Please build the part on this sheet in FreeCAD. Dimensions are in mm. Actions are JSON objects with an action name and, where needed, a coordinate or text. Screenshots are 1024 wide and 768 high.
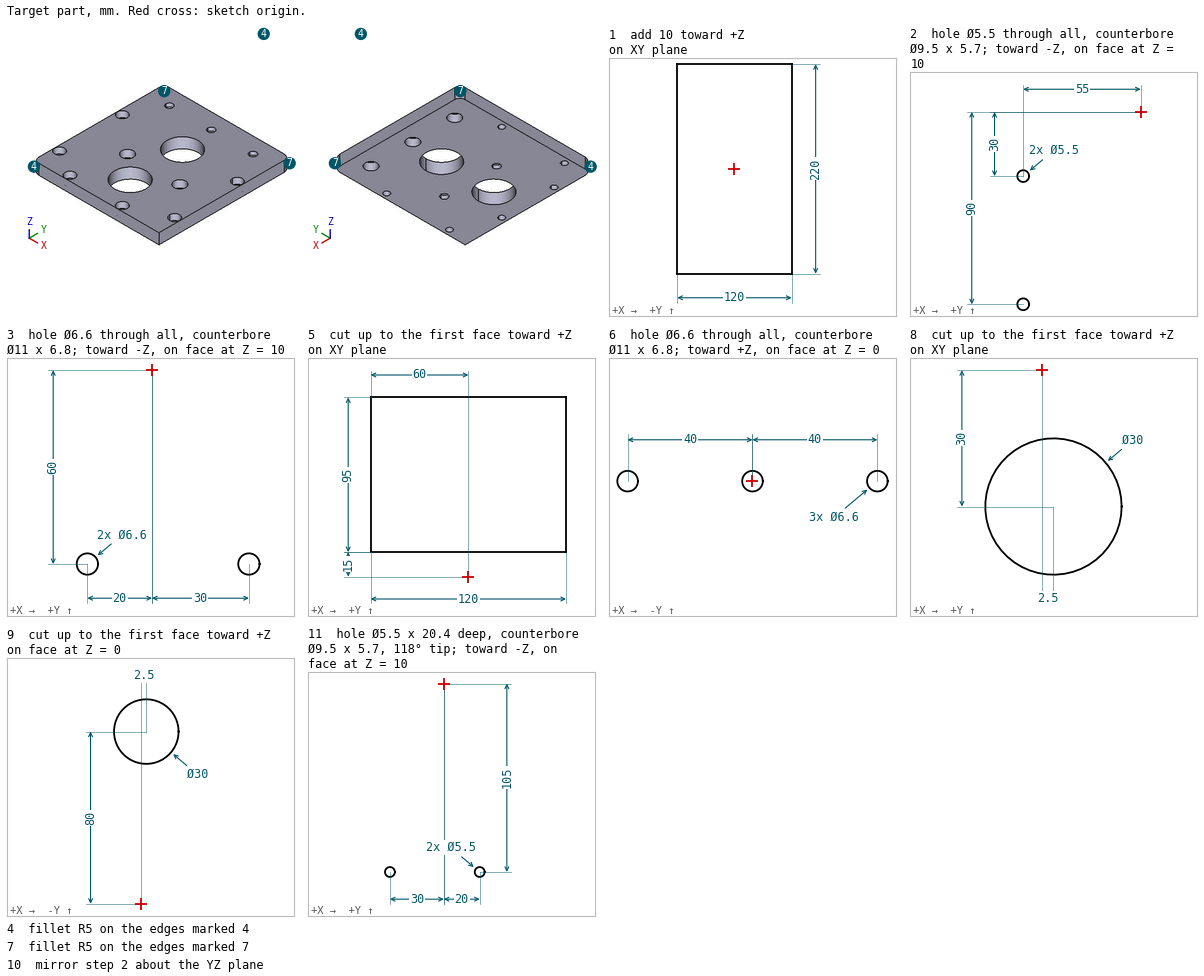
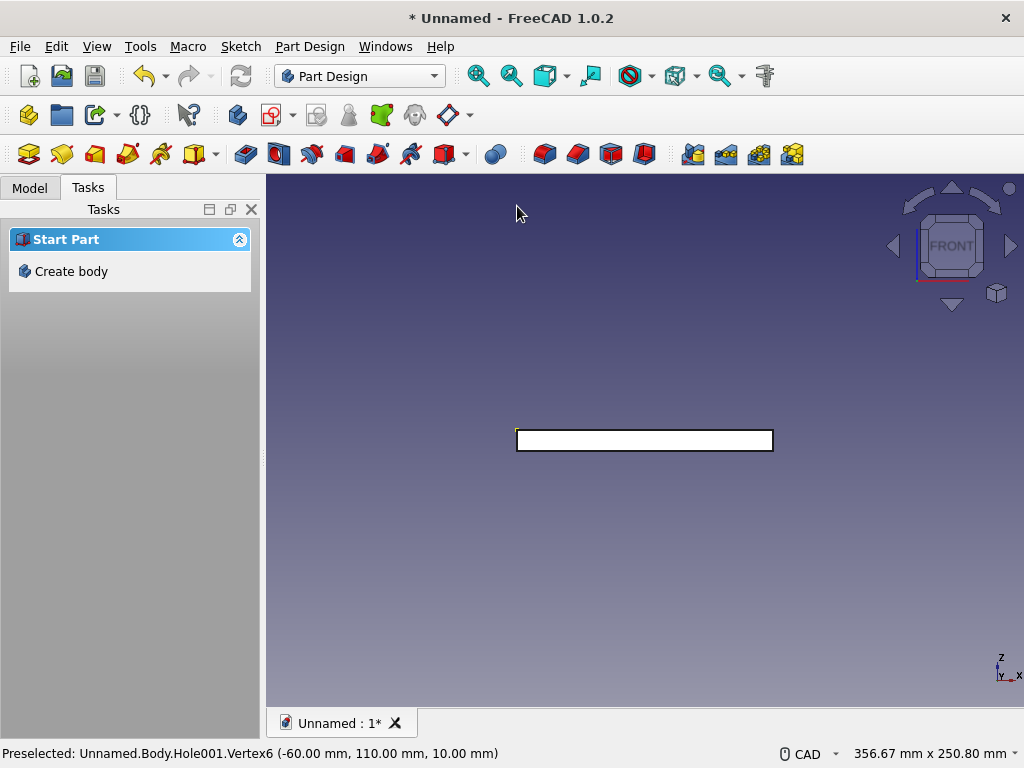
{"action": "left_click", "coordinate": [479, 76]}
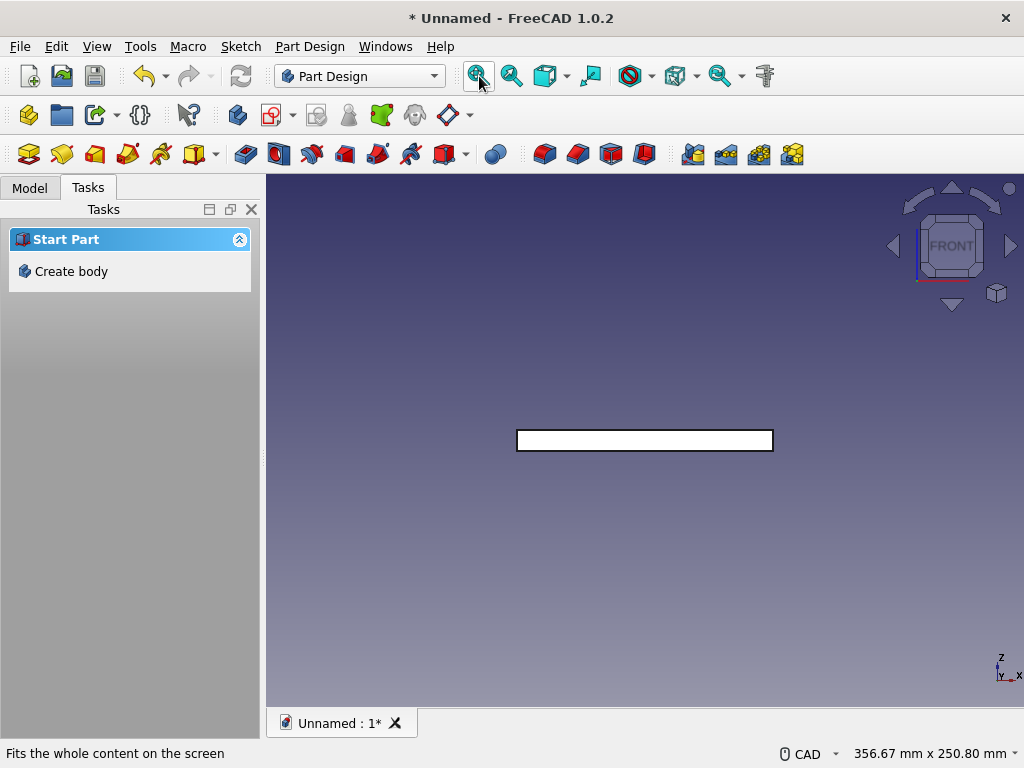
{"action": "left_click", "coordinate": [517, 440]}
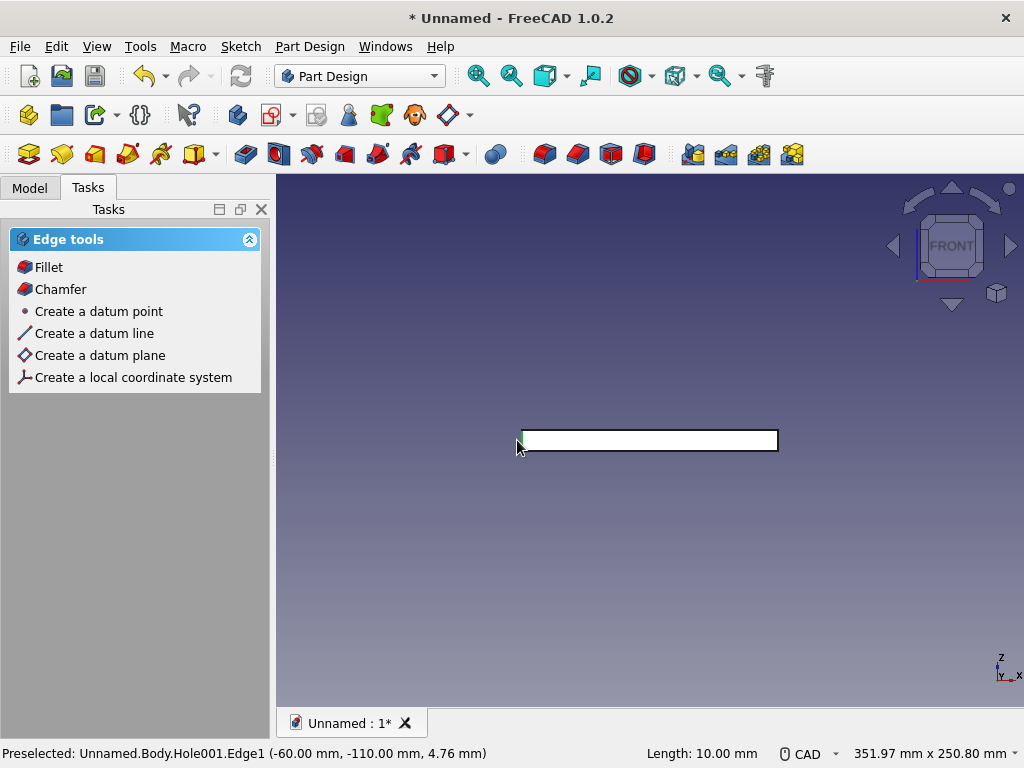
{"action": "scroll", "coordinate": [522, 440], "scroll_direction": "up", "scroll_amount": 4}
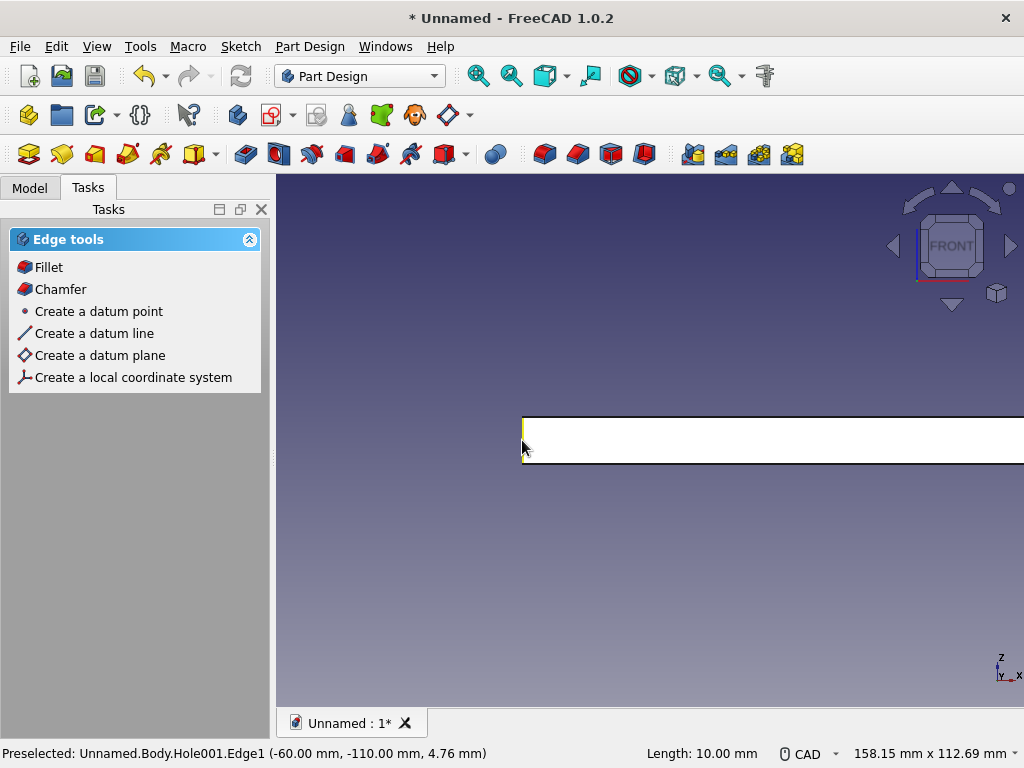
{"action": "left_click", "coordinate": [479, 76]}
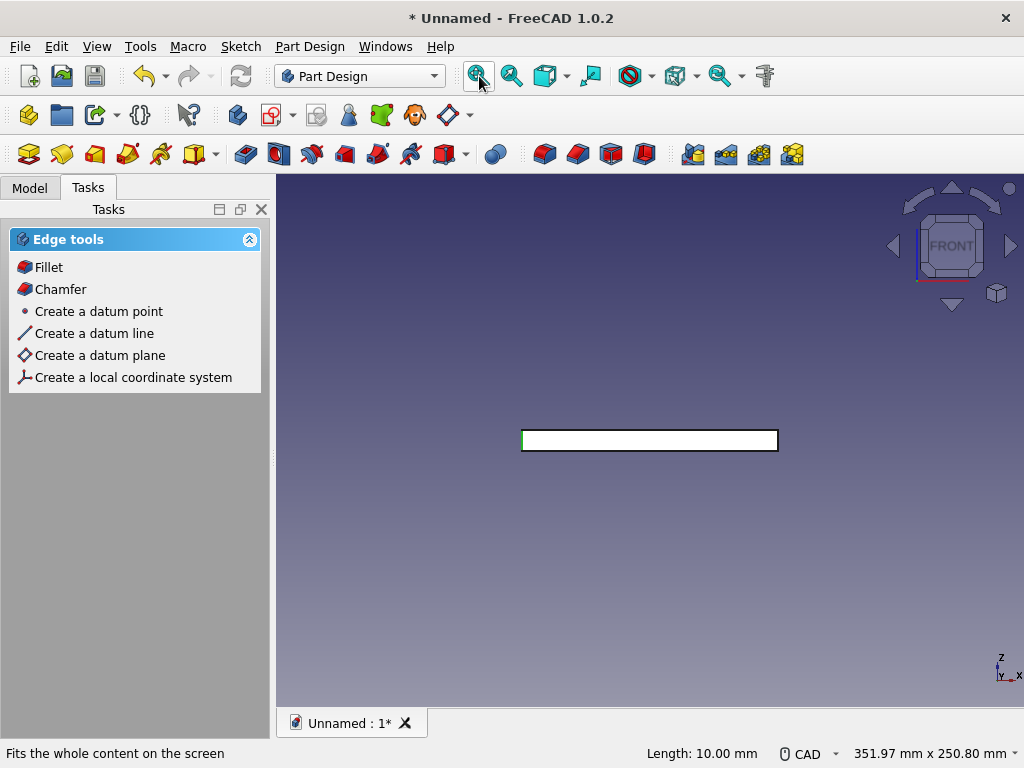
{"action": "key", "text": "3"}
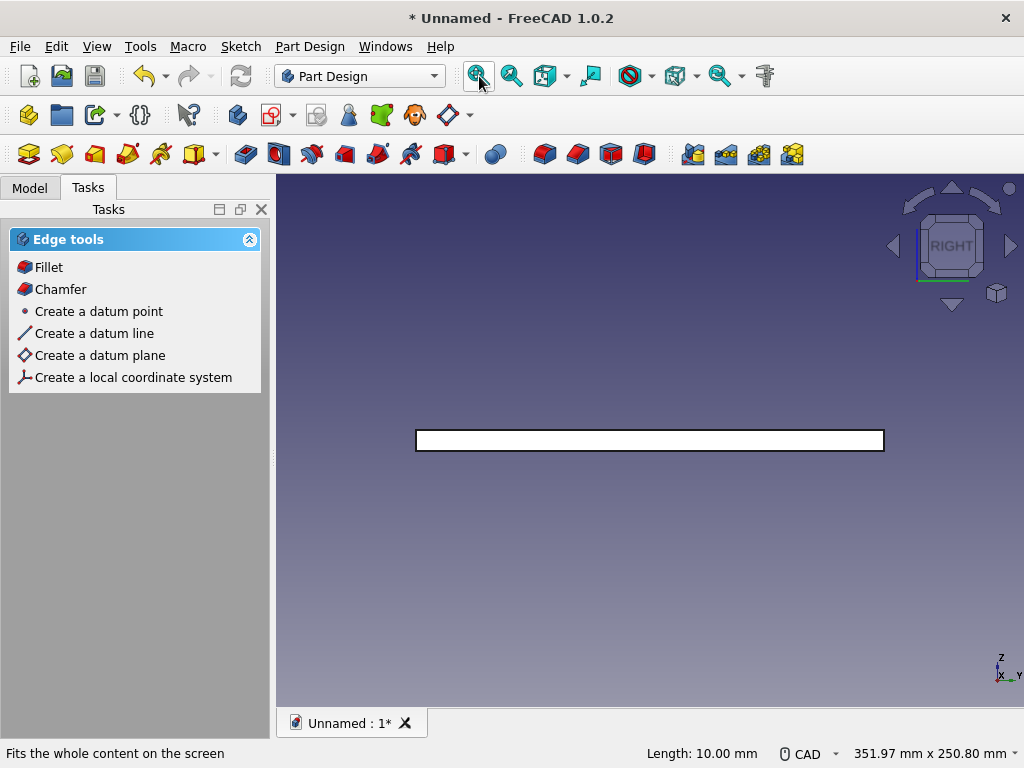
{"action": "key", "text": "5"}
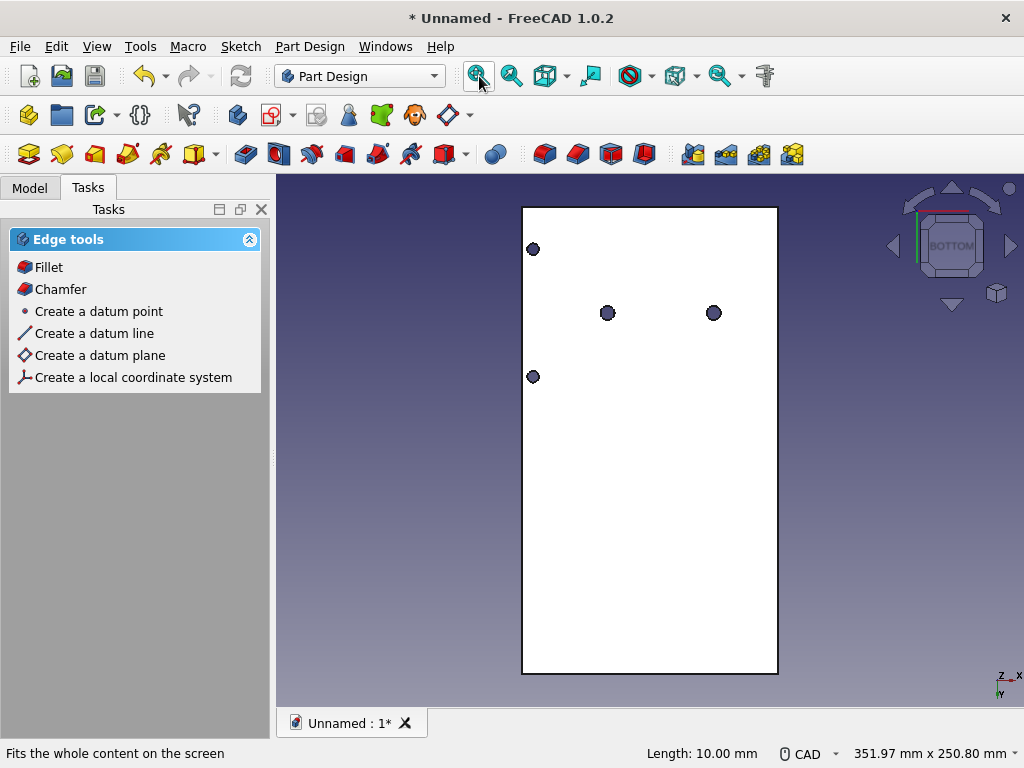
{"action": "scroll", "coordinate": [522, 673], "scroll_direction": "up", "scroll_amount": 4}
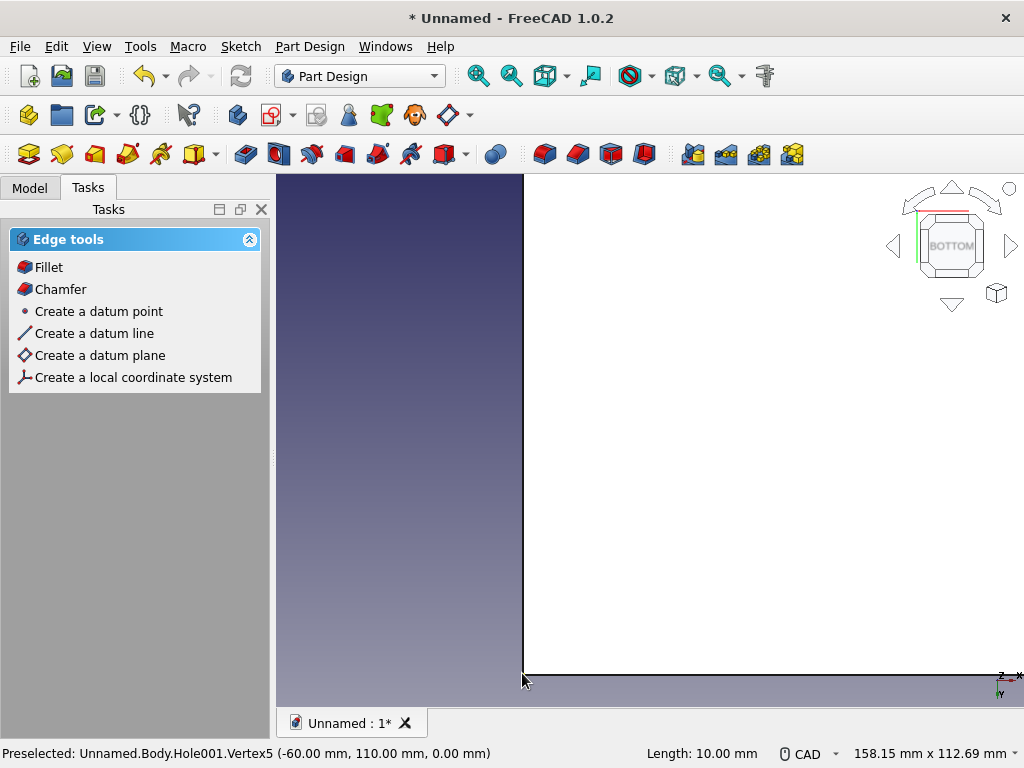
{"action": "left_click", "coordinate": [479, 76]}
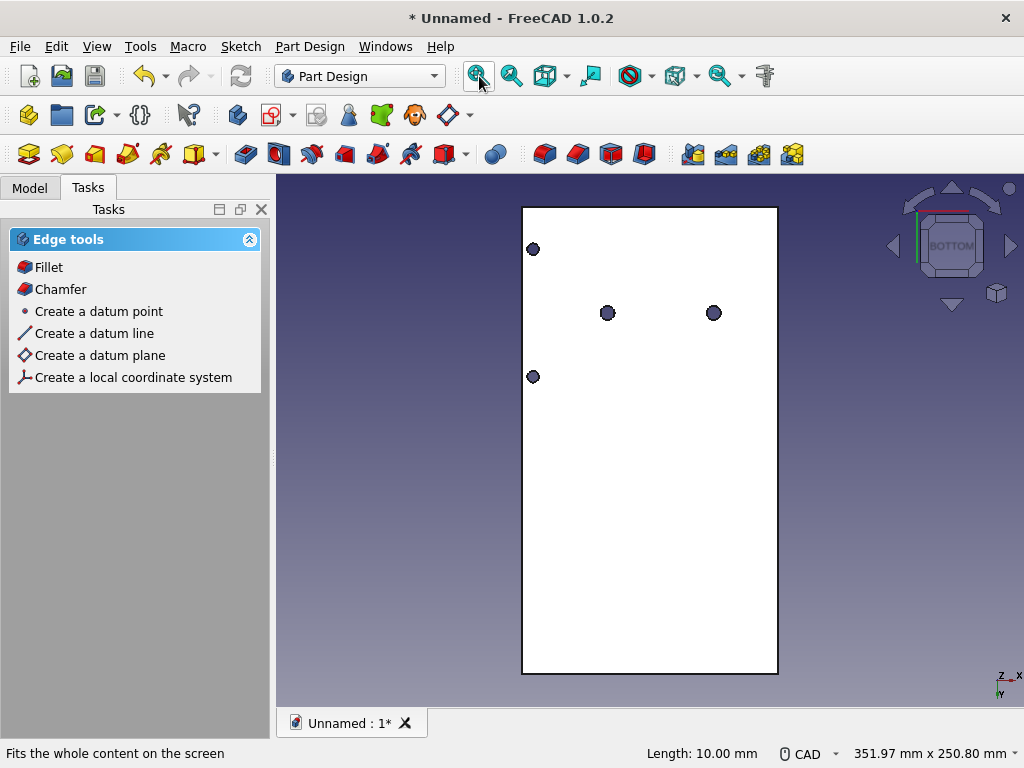
{"action": "key", "text": "4"}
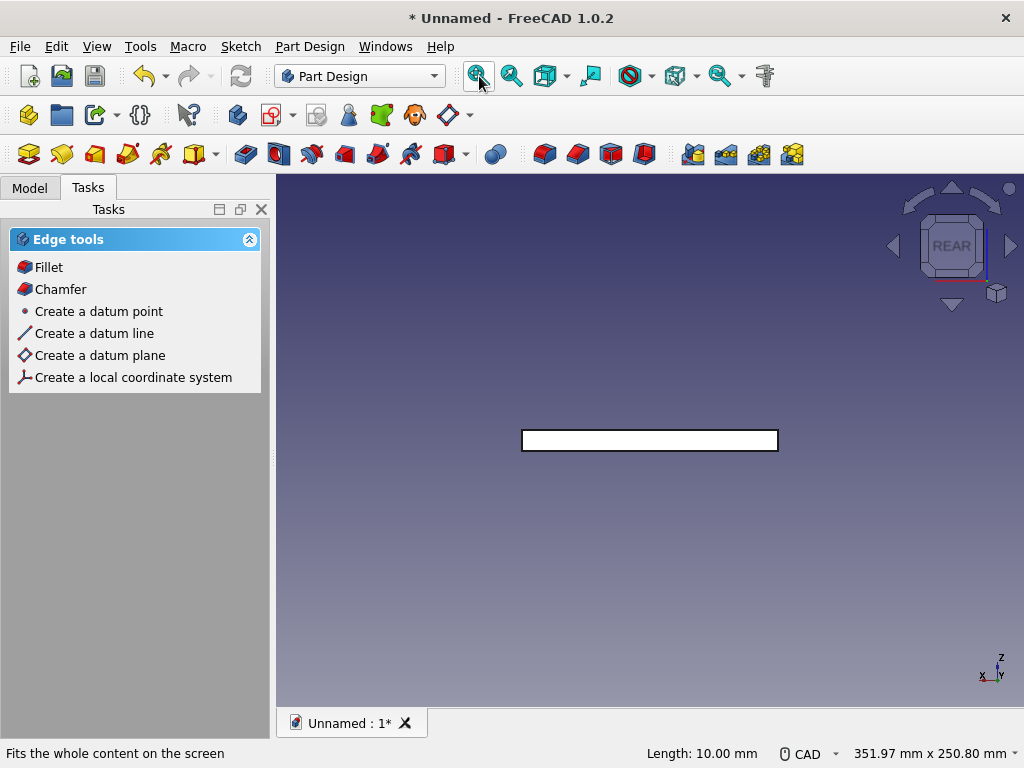
{"action": "left_click", "coordinate": [479, 76]}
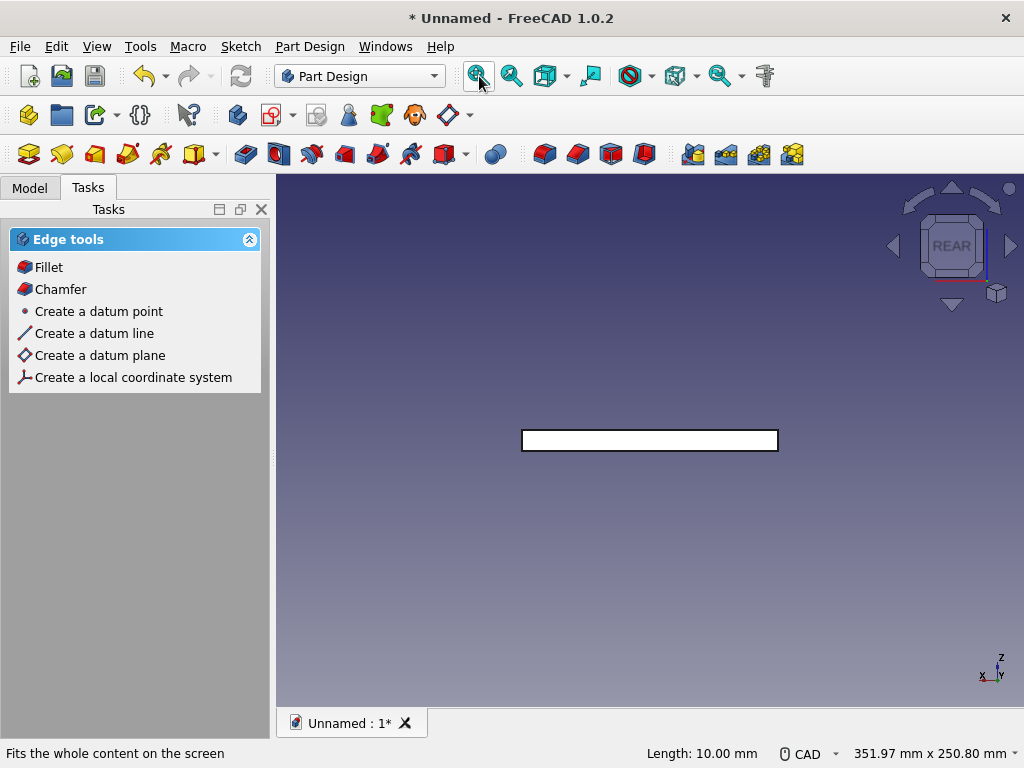
{"action": "left_click", "coordinate": [778, 440], "text": "ctrl"}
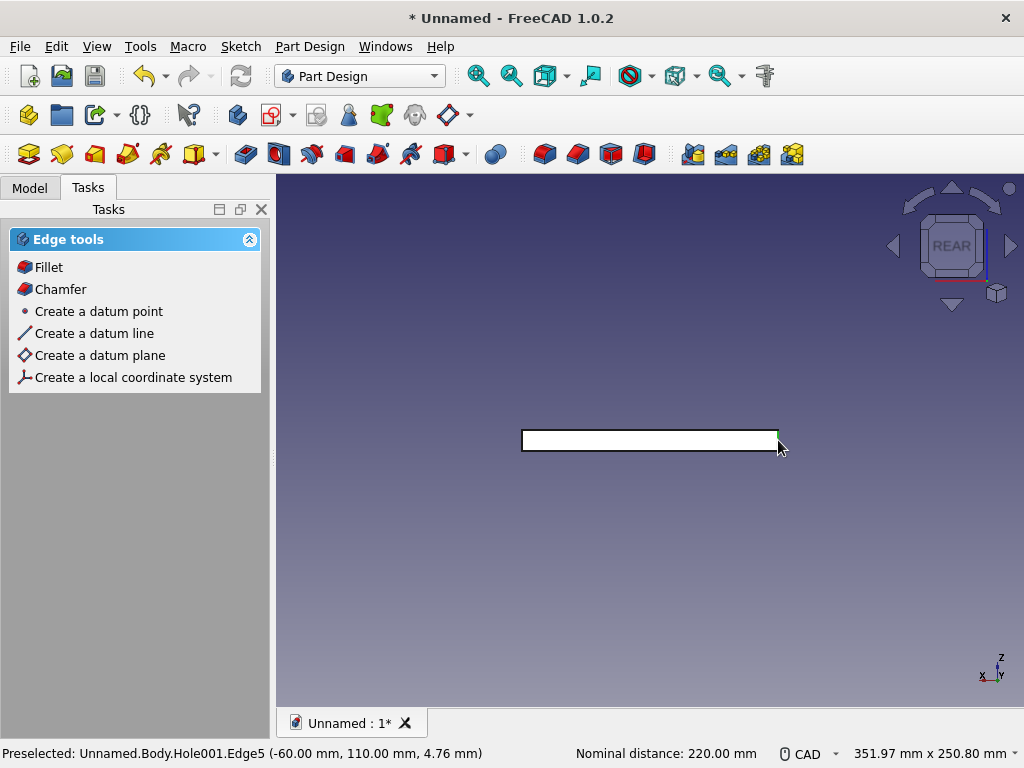
{"action": "left_click", "coordinate": [545, 154]}